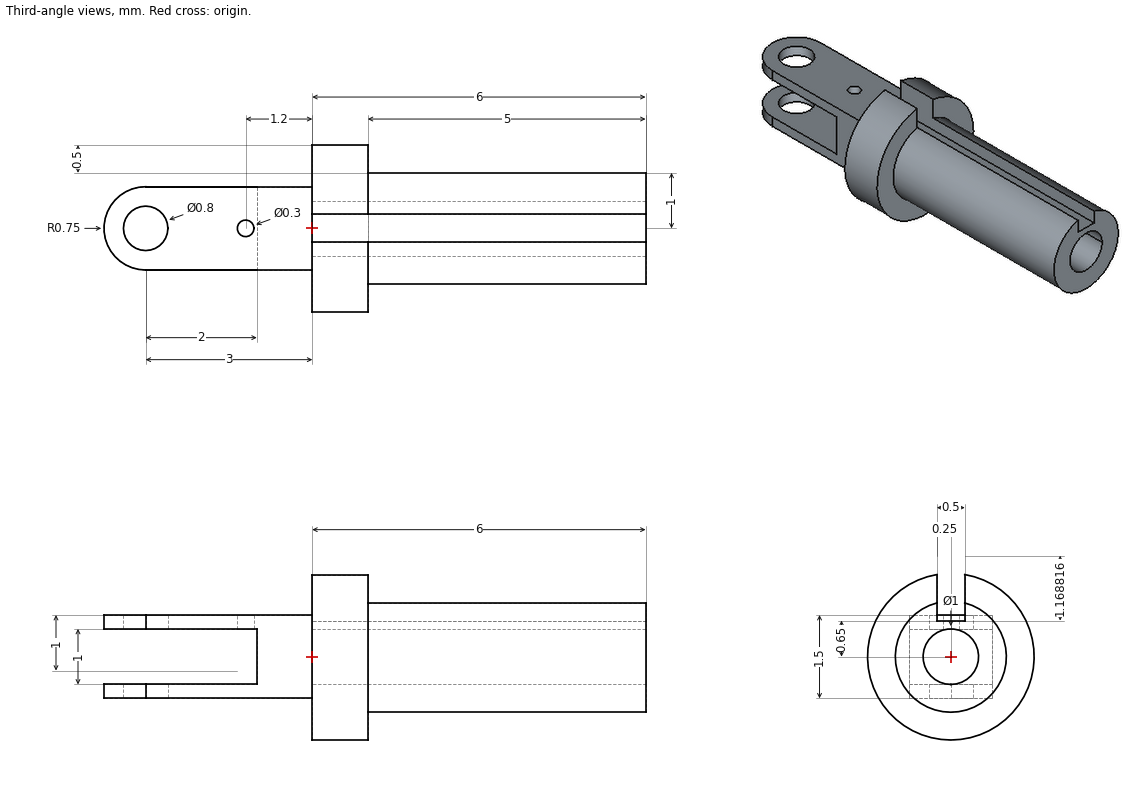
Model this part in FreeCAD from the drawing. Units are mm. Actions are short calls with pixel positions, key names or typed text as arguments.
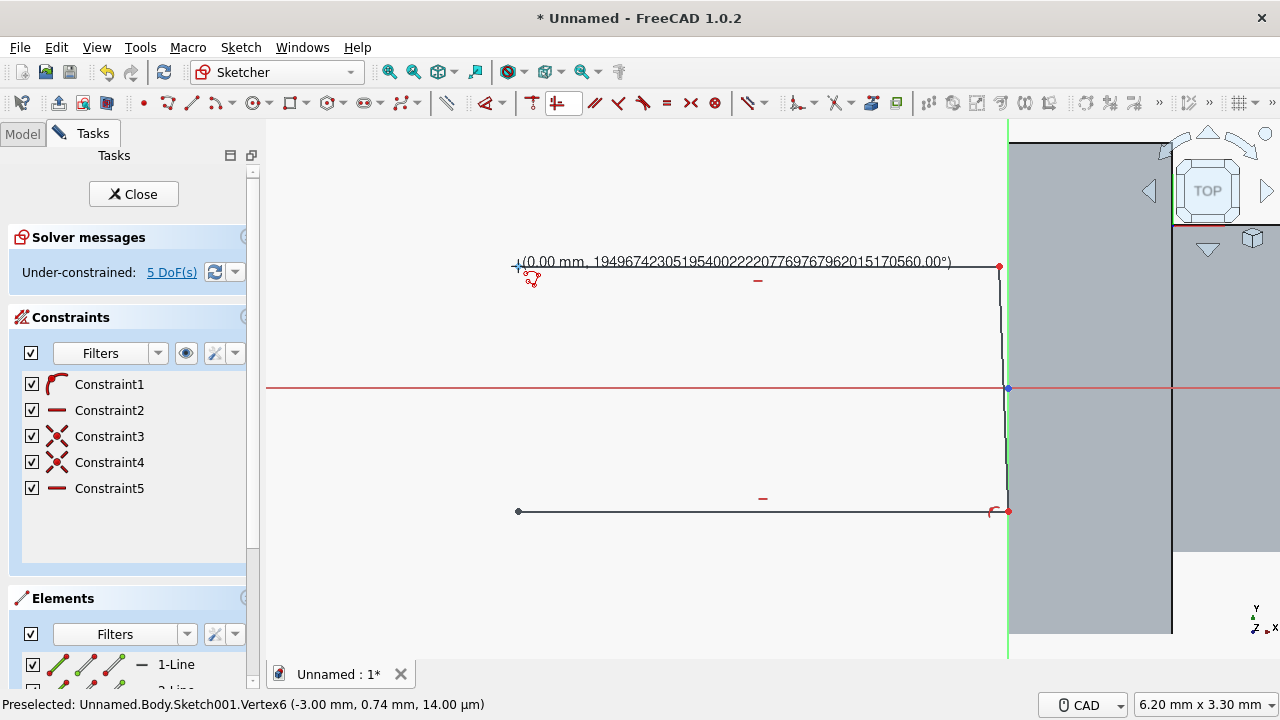
click(234, 104)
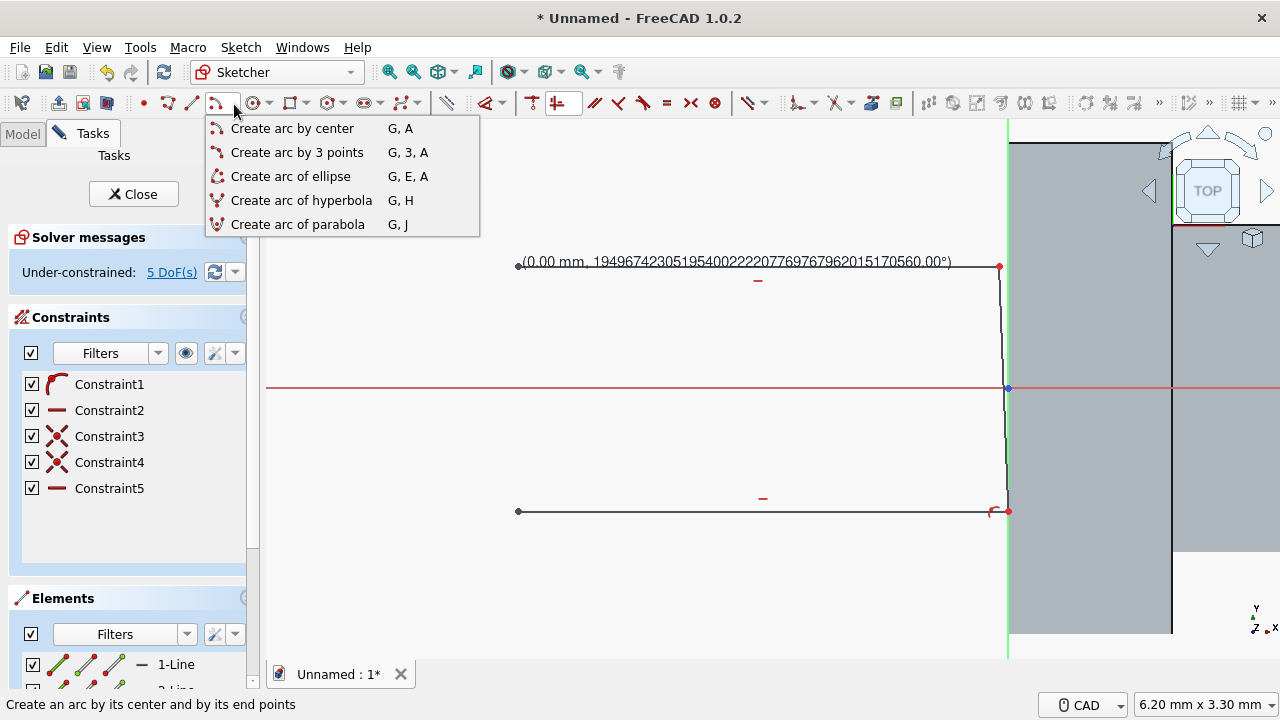
click(342, 152)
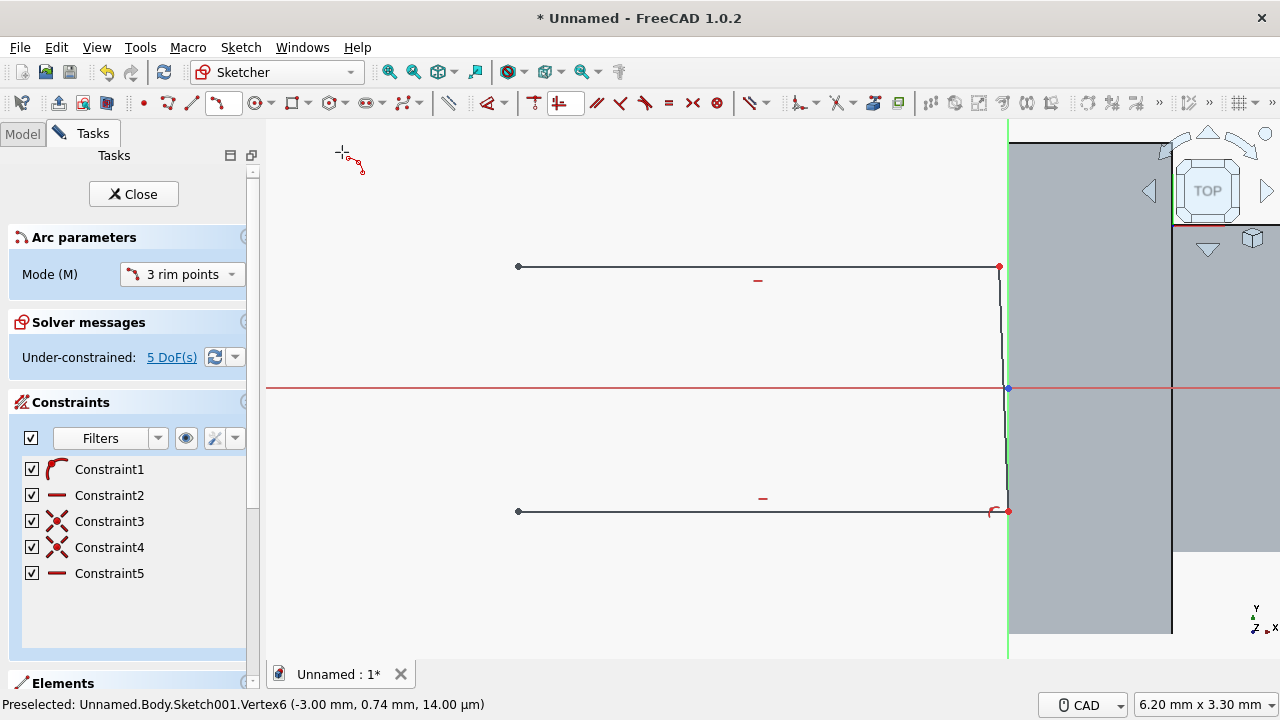
click(518, 267)
click(518, 512)
click(401, 350)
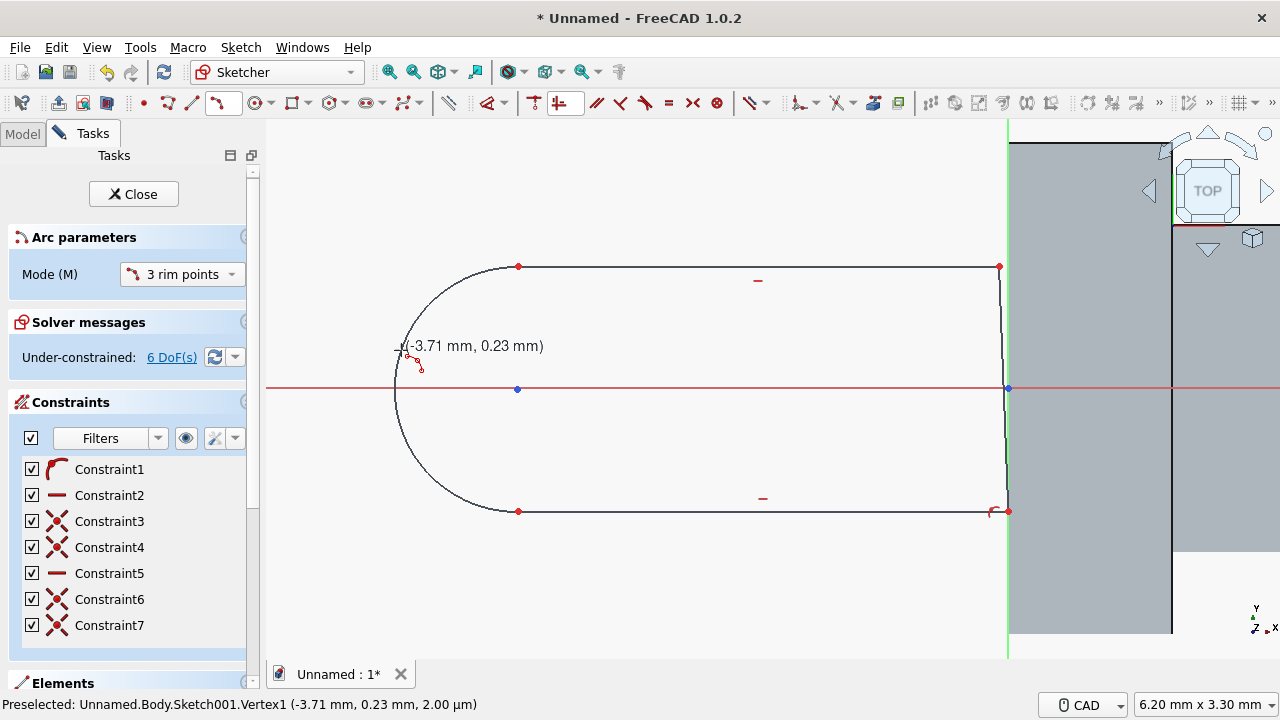
click(256, 104)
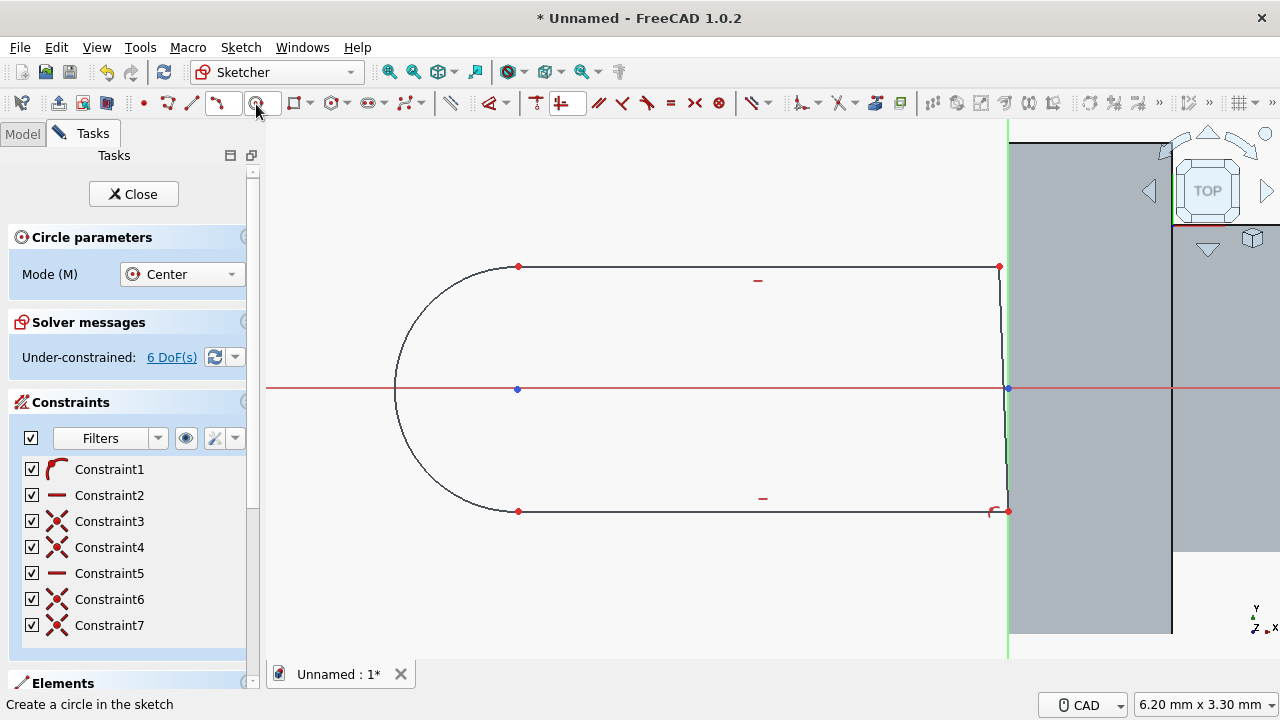
click(518, 388)
move(564, 342)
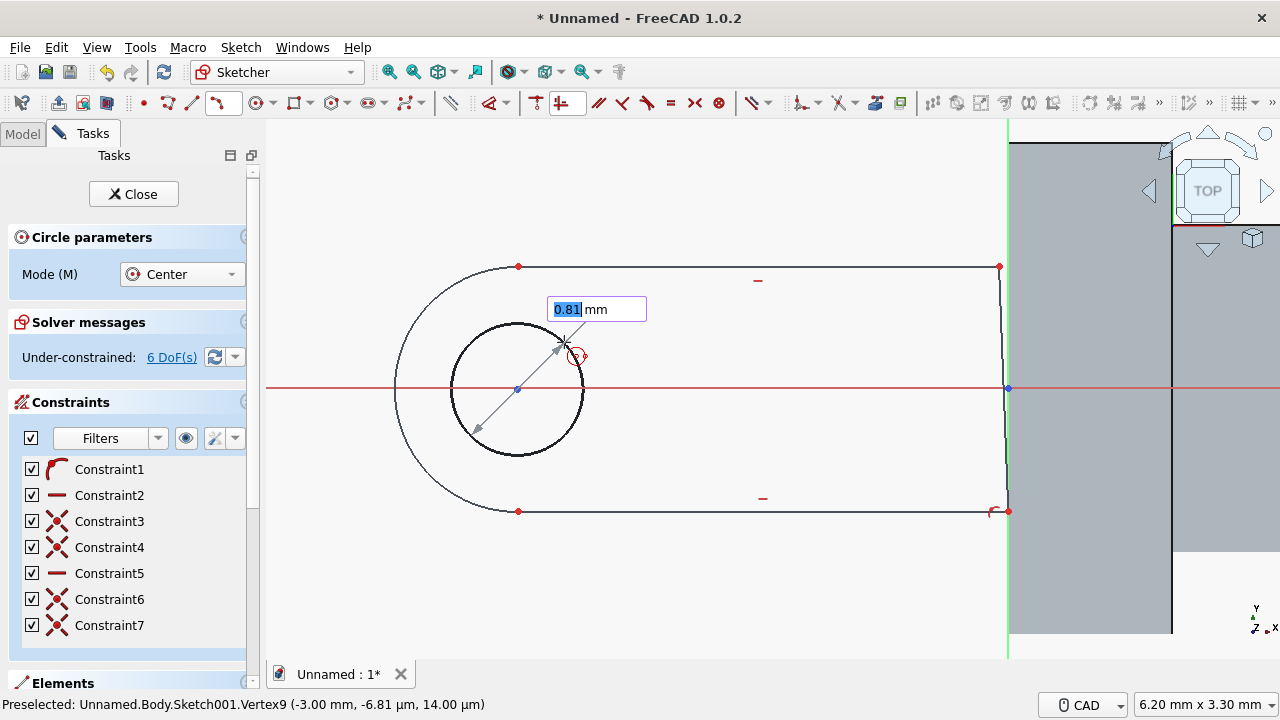
text(0.8)
key(Return)
key(Escape)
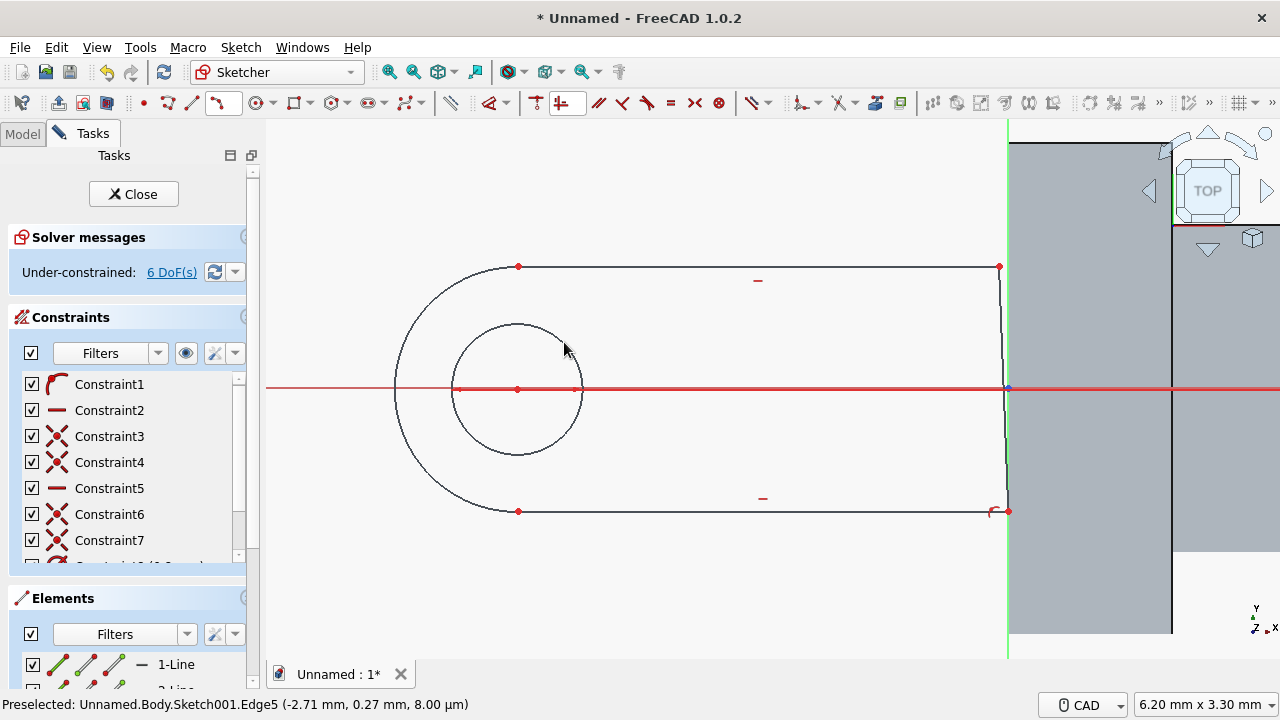
click(665, 512)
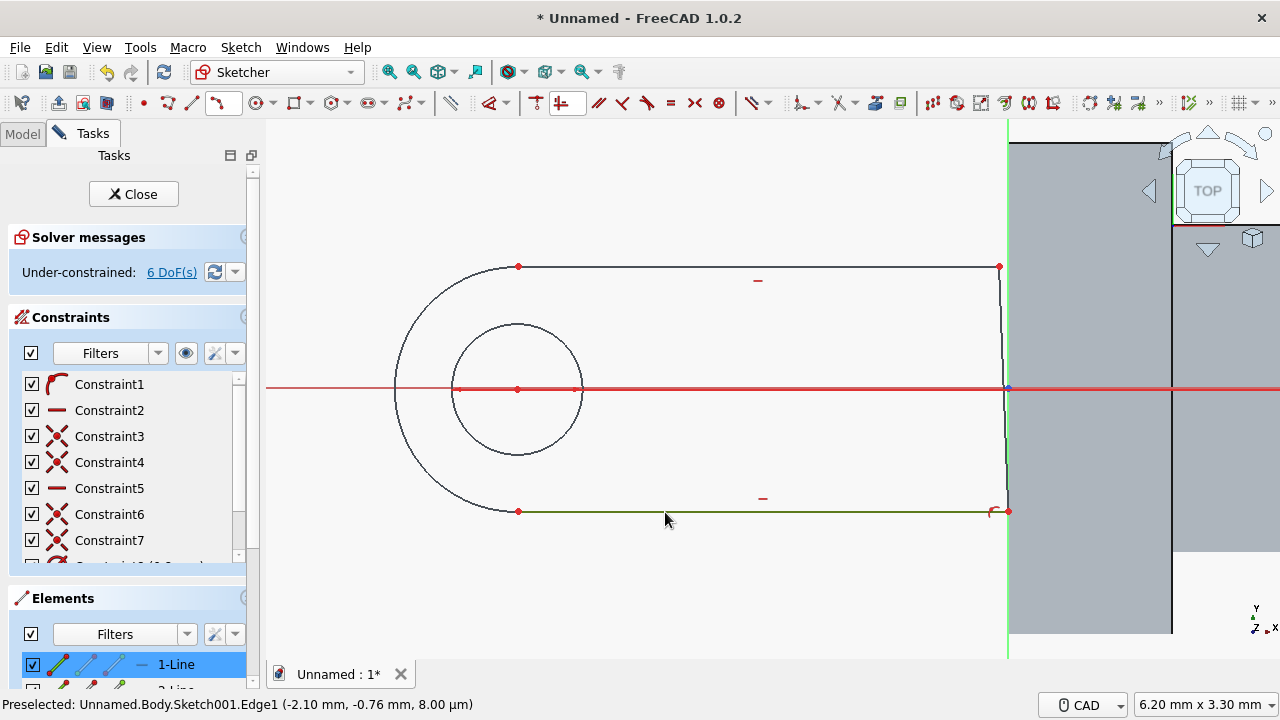
click(418, 317)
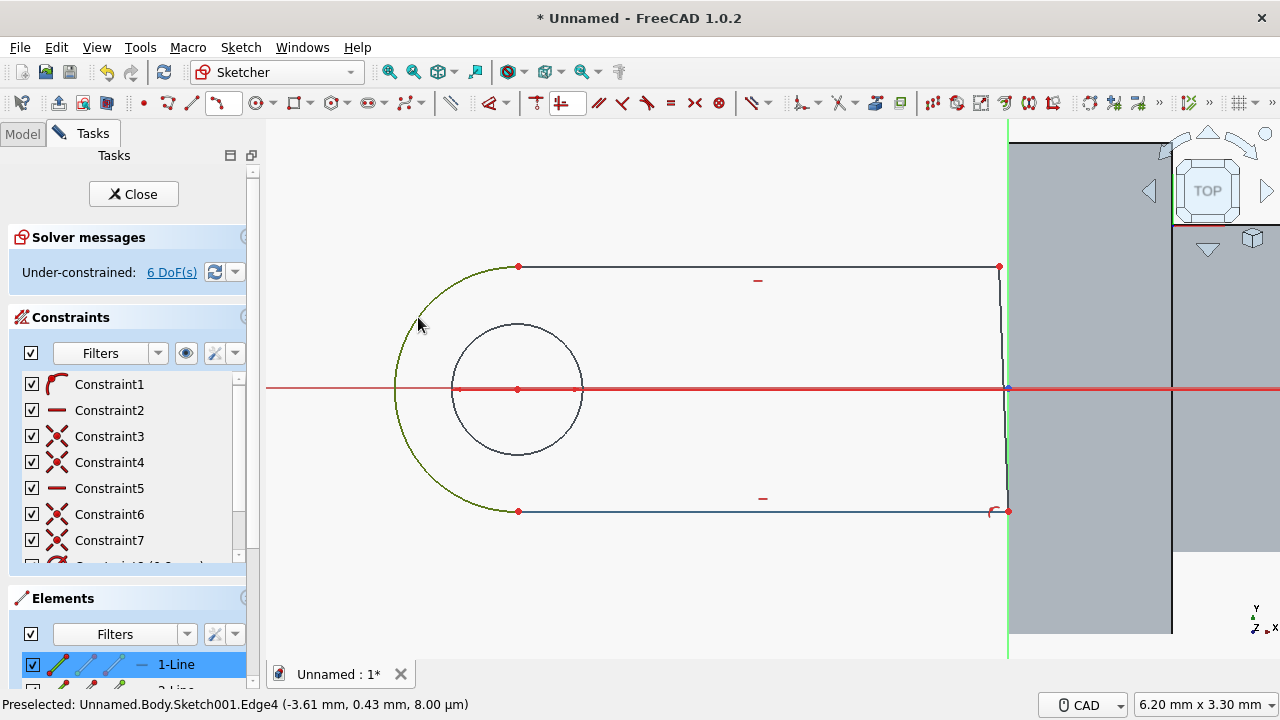
click(648, 104)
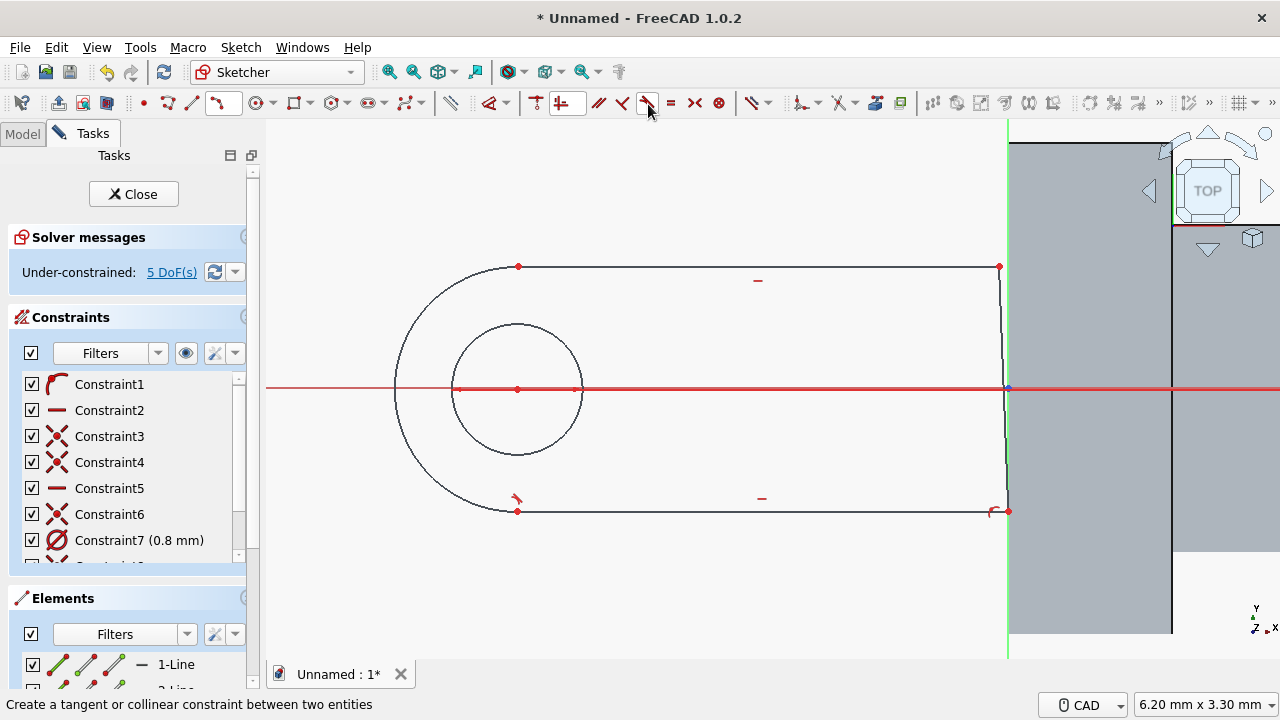
click(855, 267)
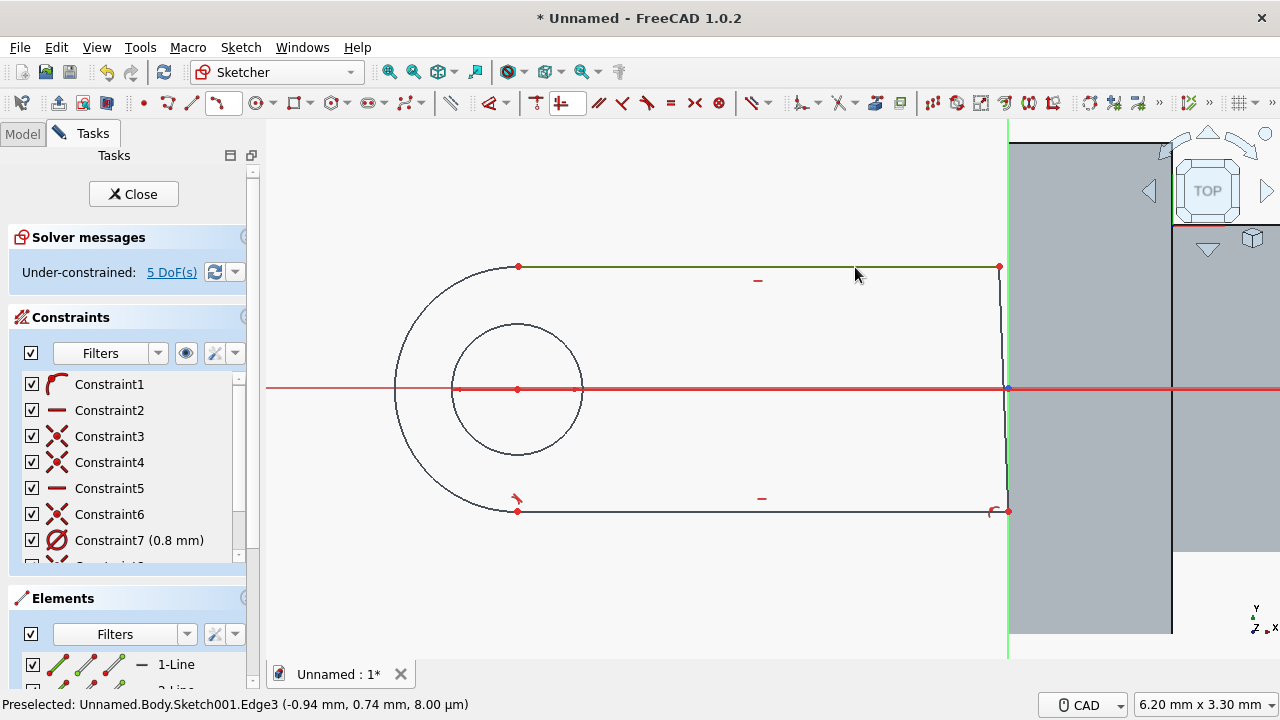
click(418, 317)